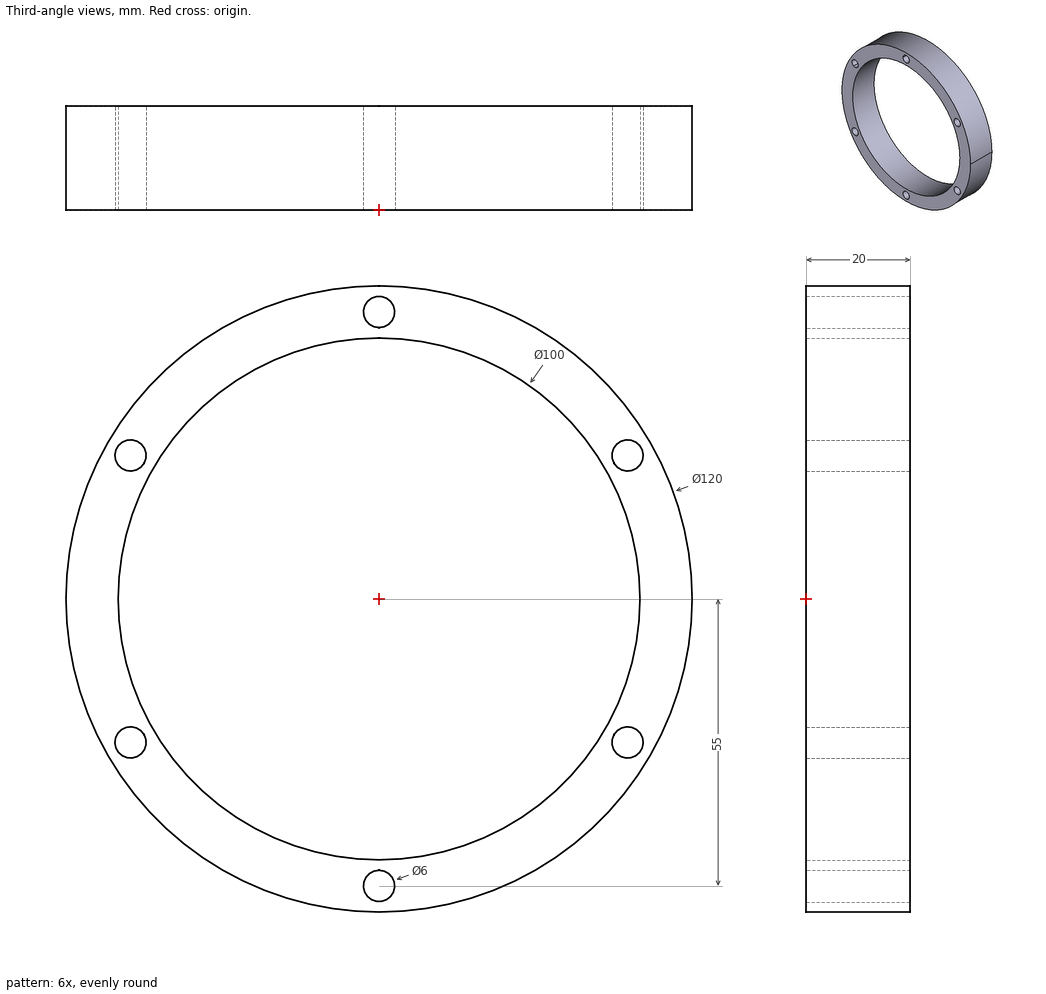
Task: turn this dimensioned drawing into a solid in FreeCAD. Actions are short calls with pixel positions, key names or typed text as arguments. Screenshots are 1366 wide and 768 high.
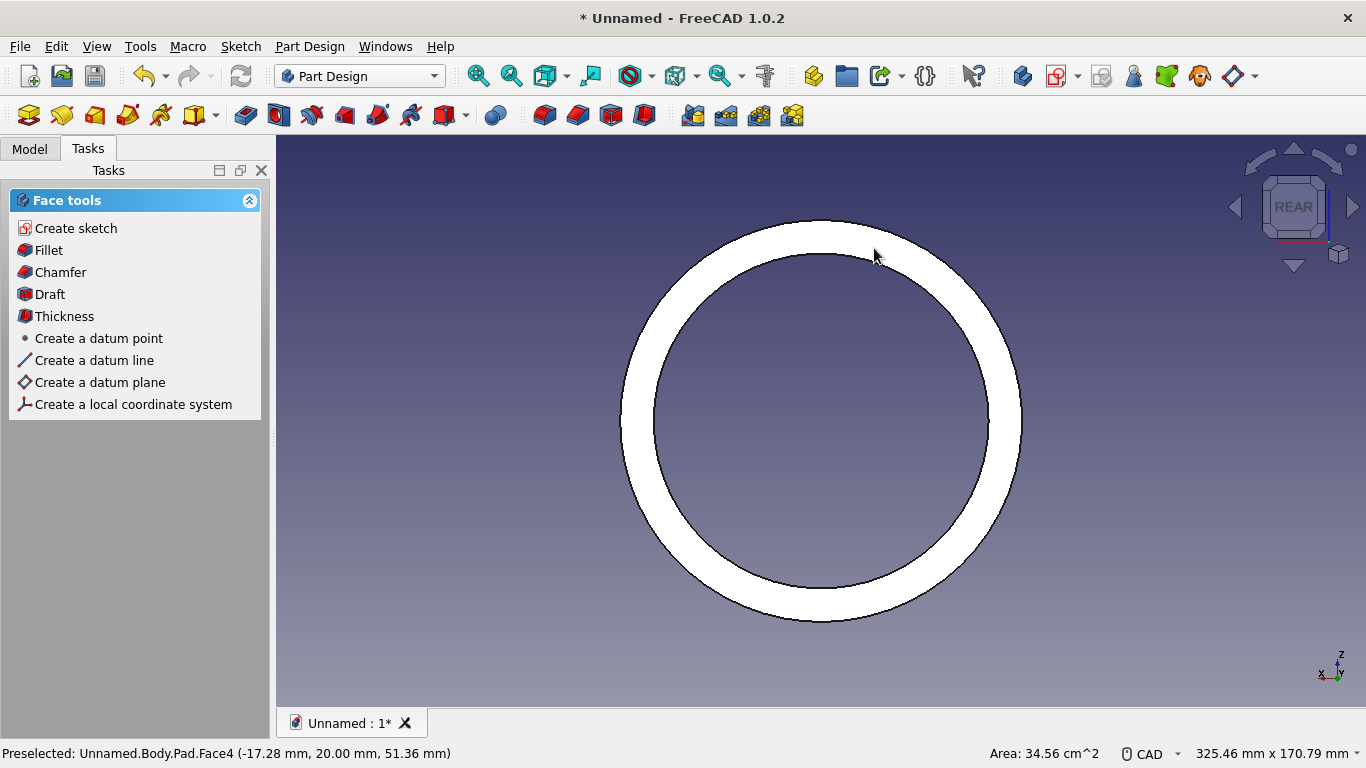
click(1056, 76)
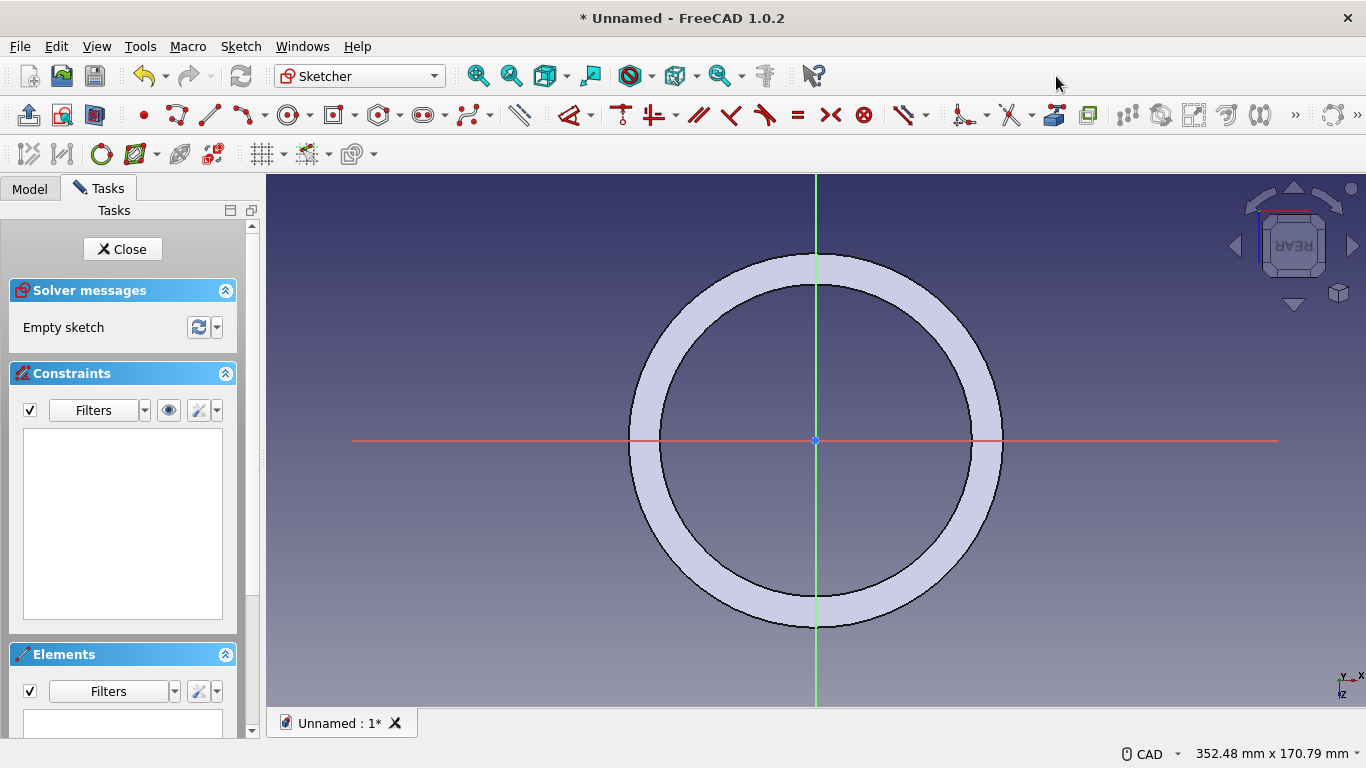
scroll(820, 258, up, 14)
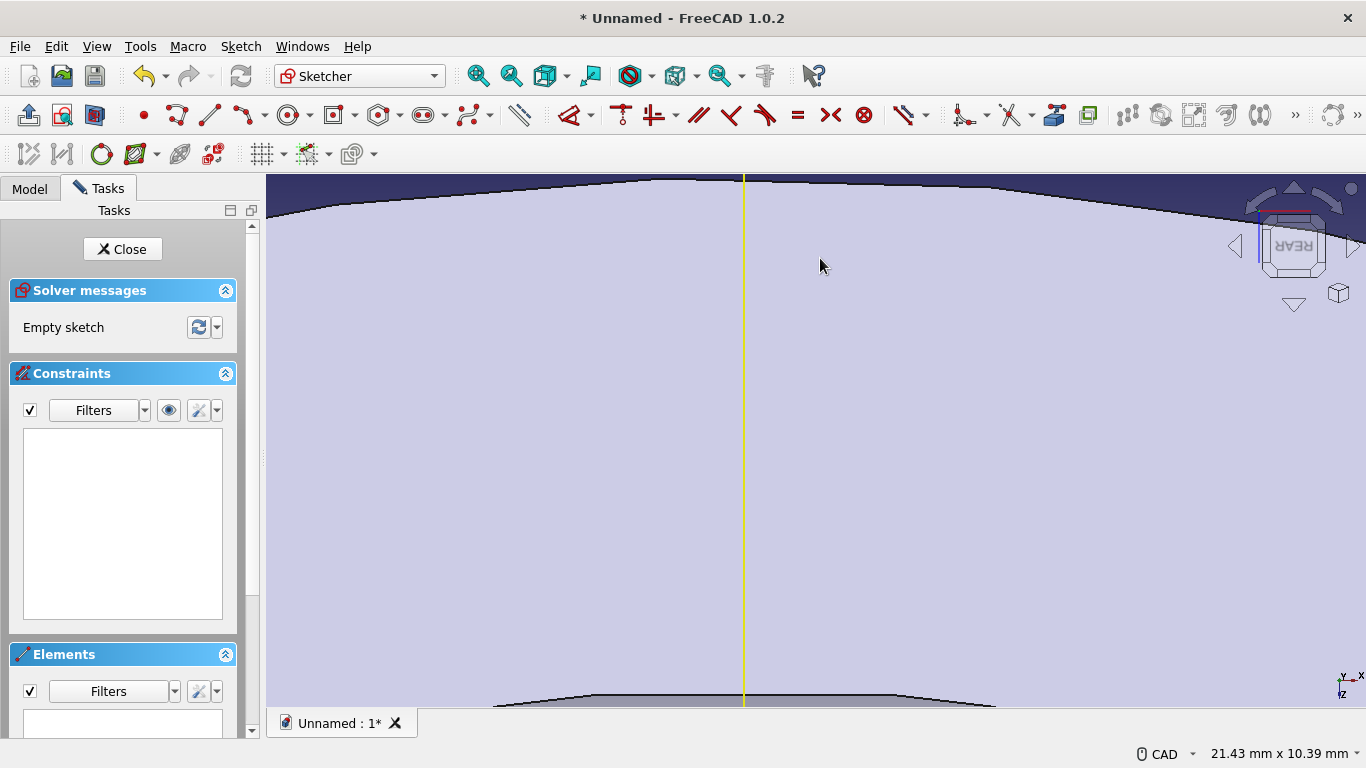
key(g)
key(c)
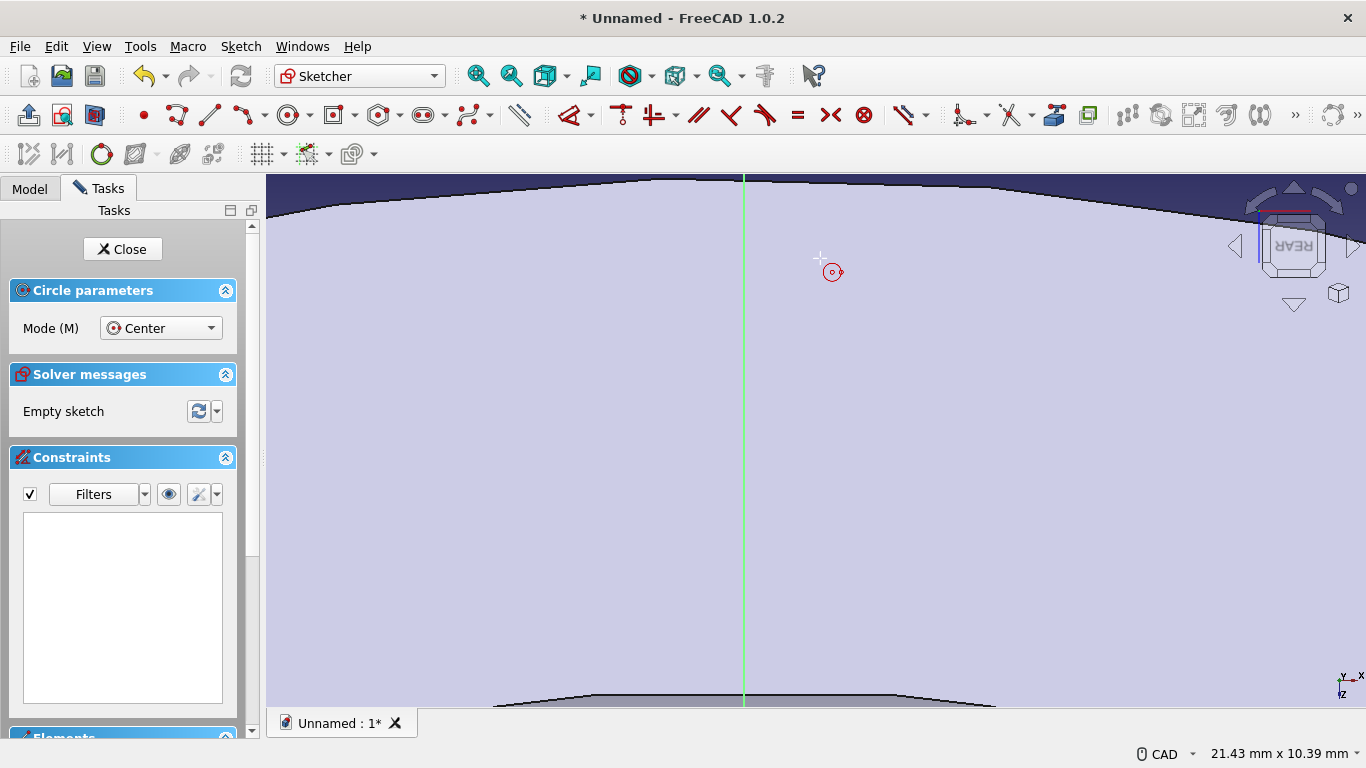
click(744, 434)
move(853, 325)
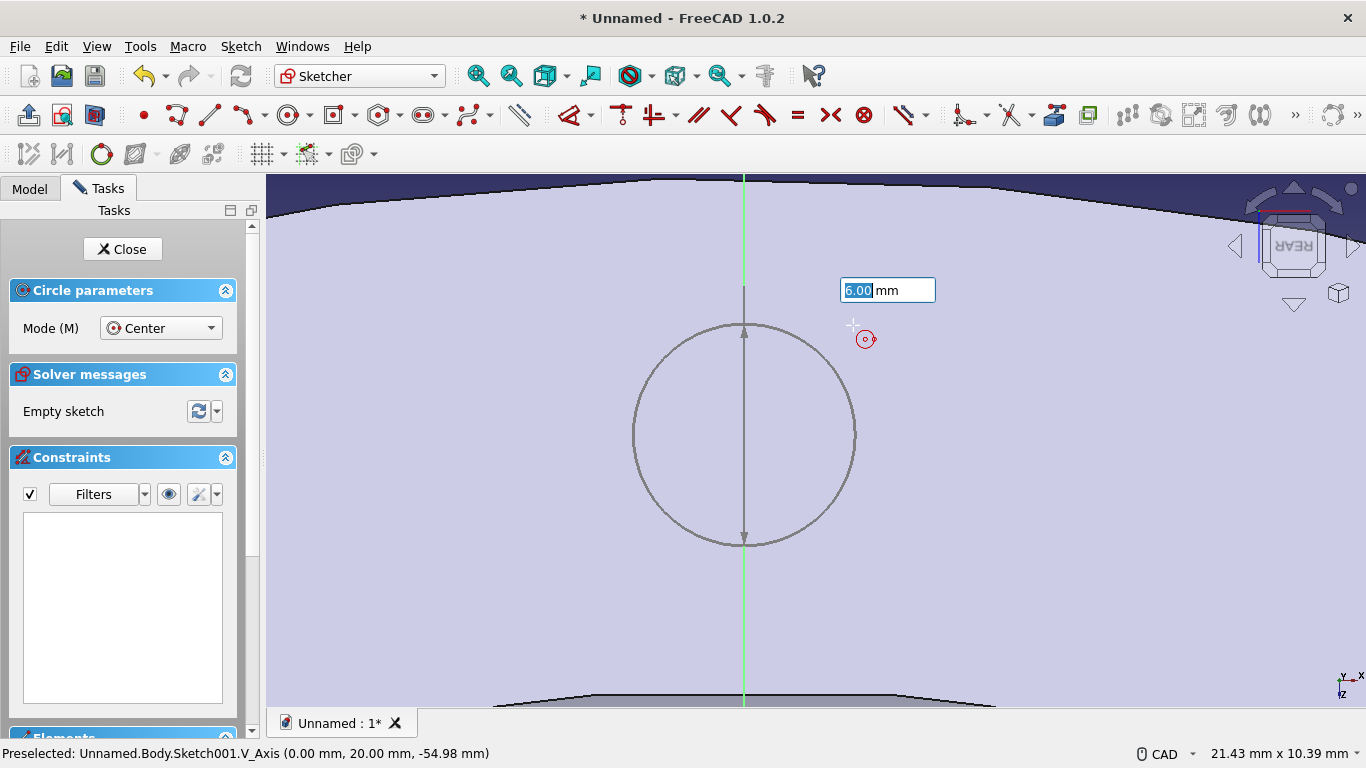
text(6)
key(Return)
key(Escape)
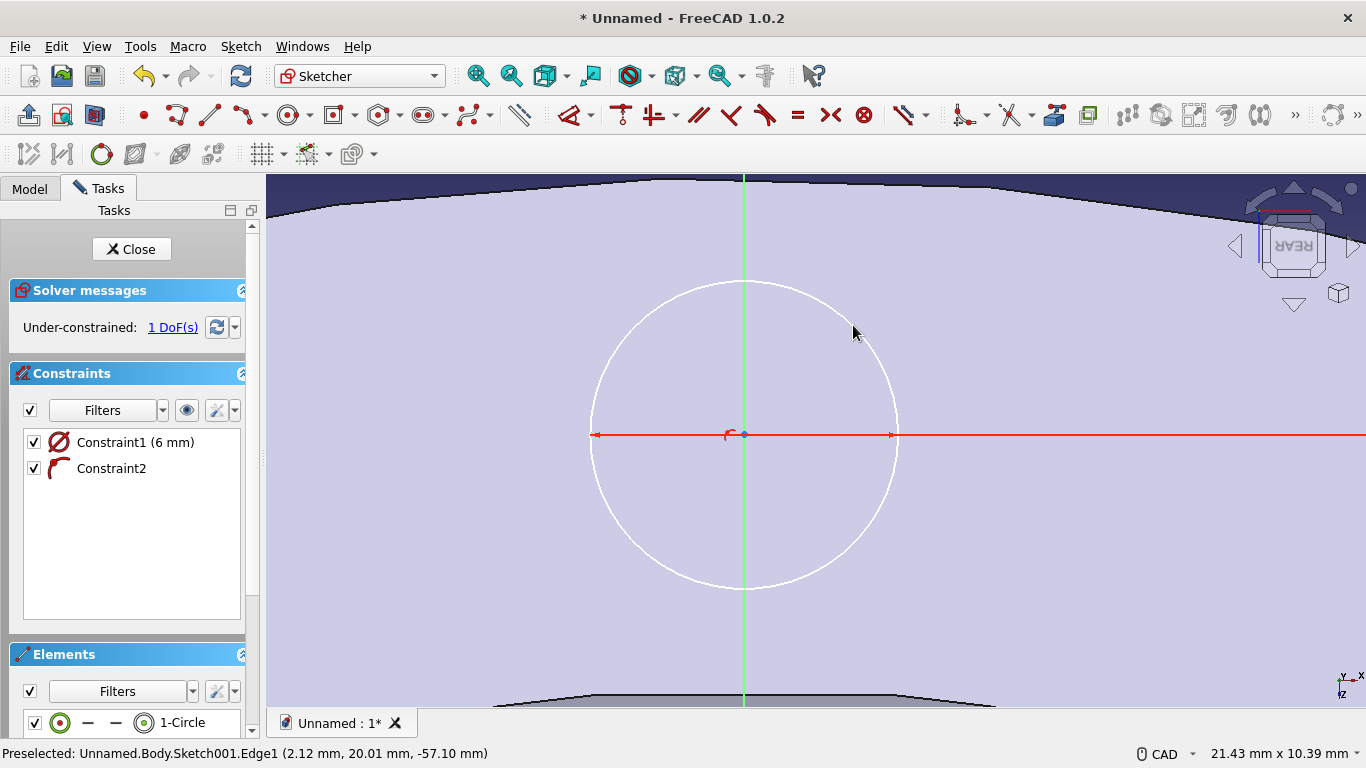
click(744, 435)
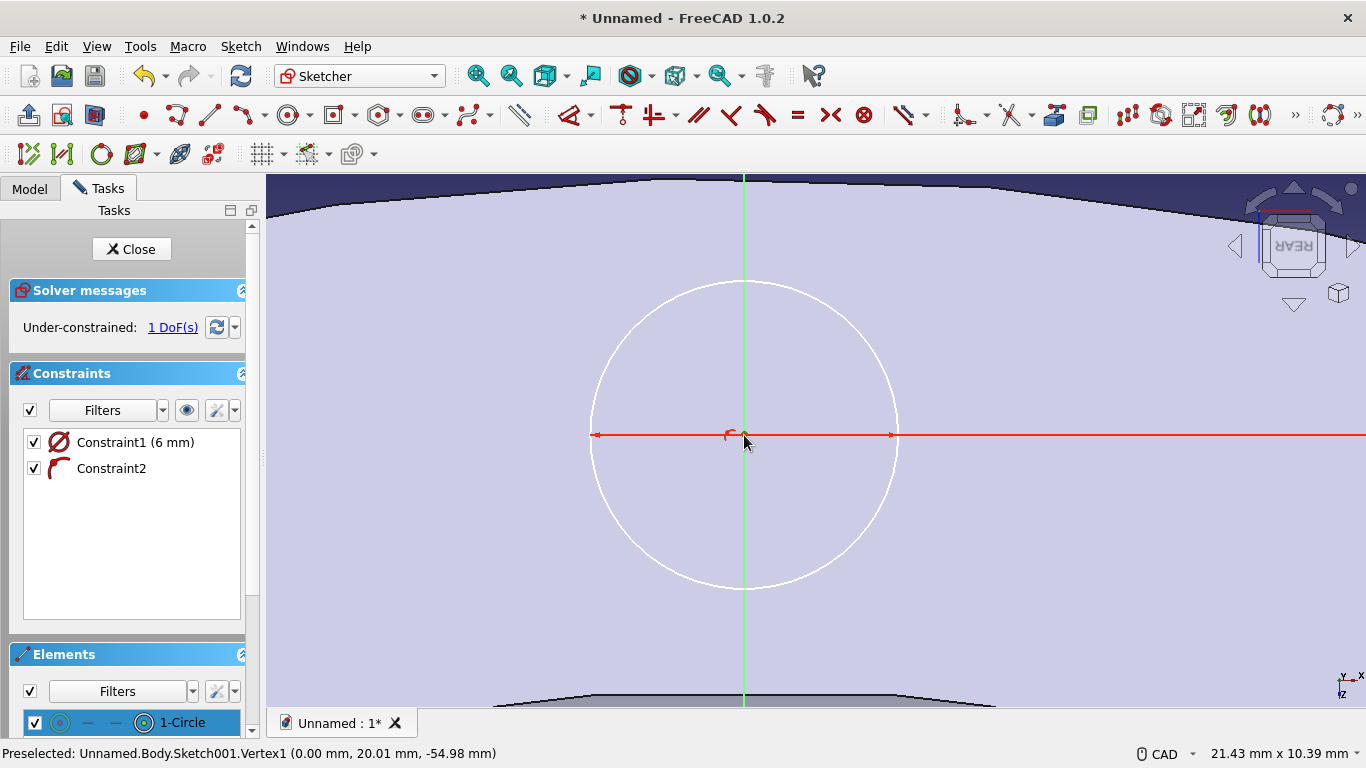
key(i)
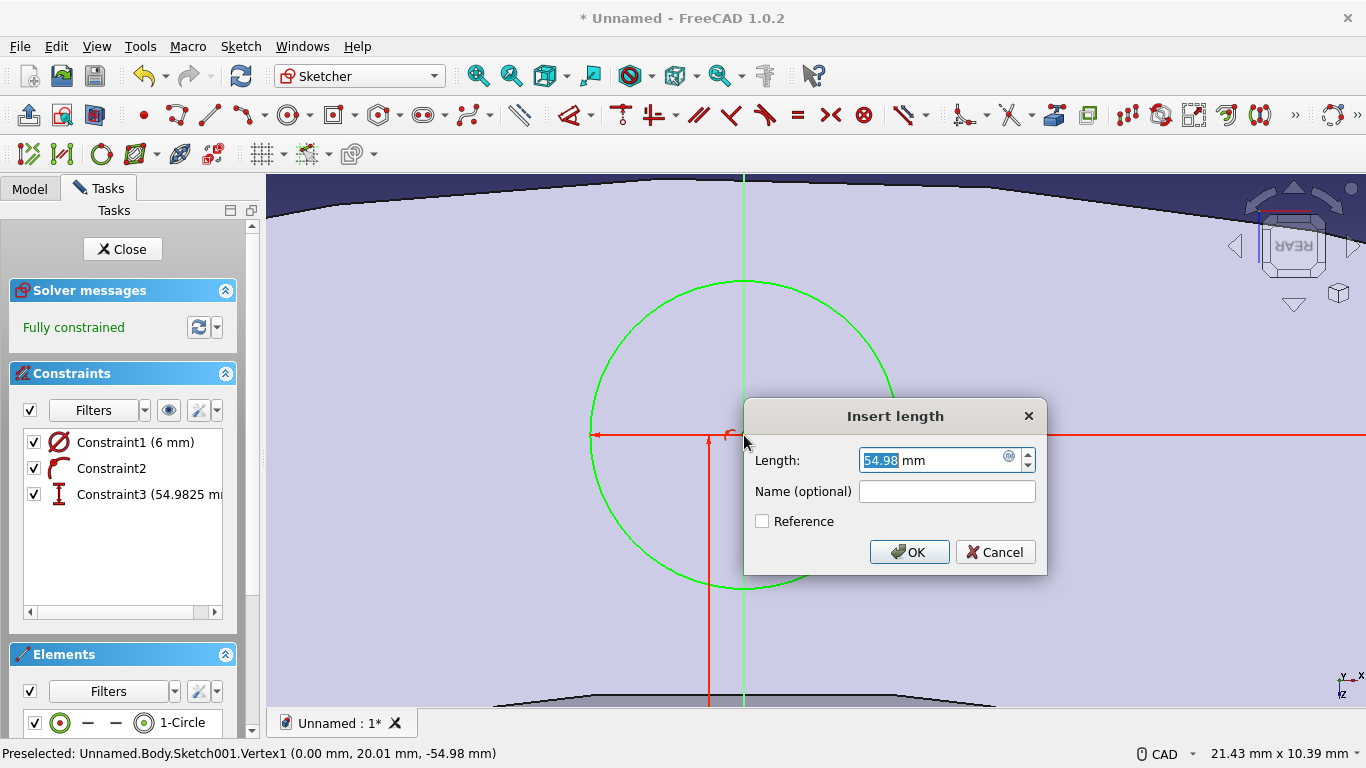
text(55)
key(Return)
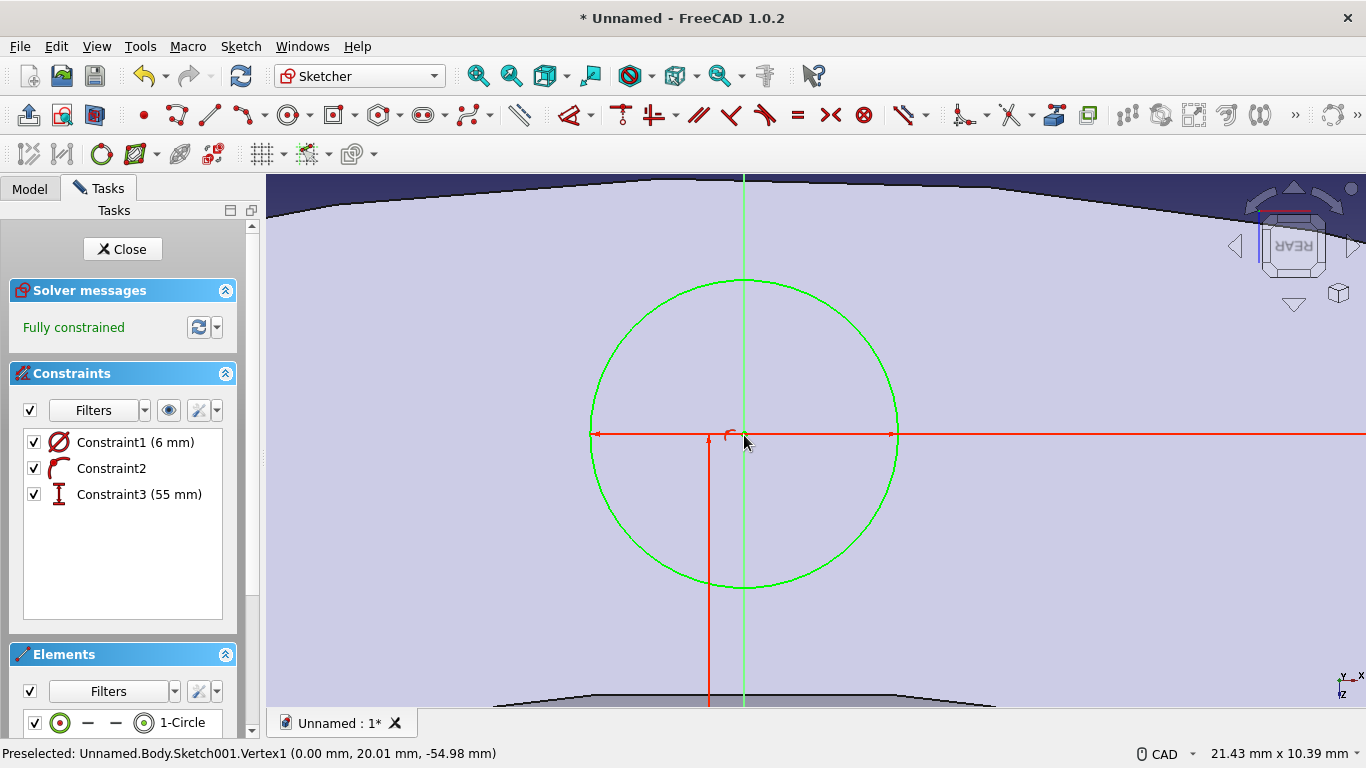
click(123, 249)